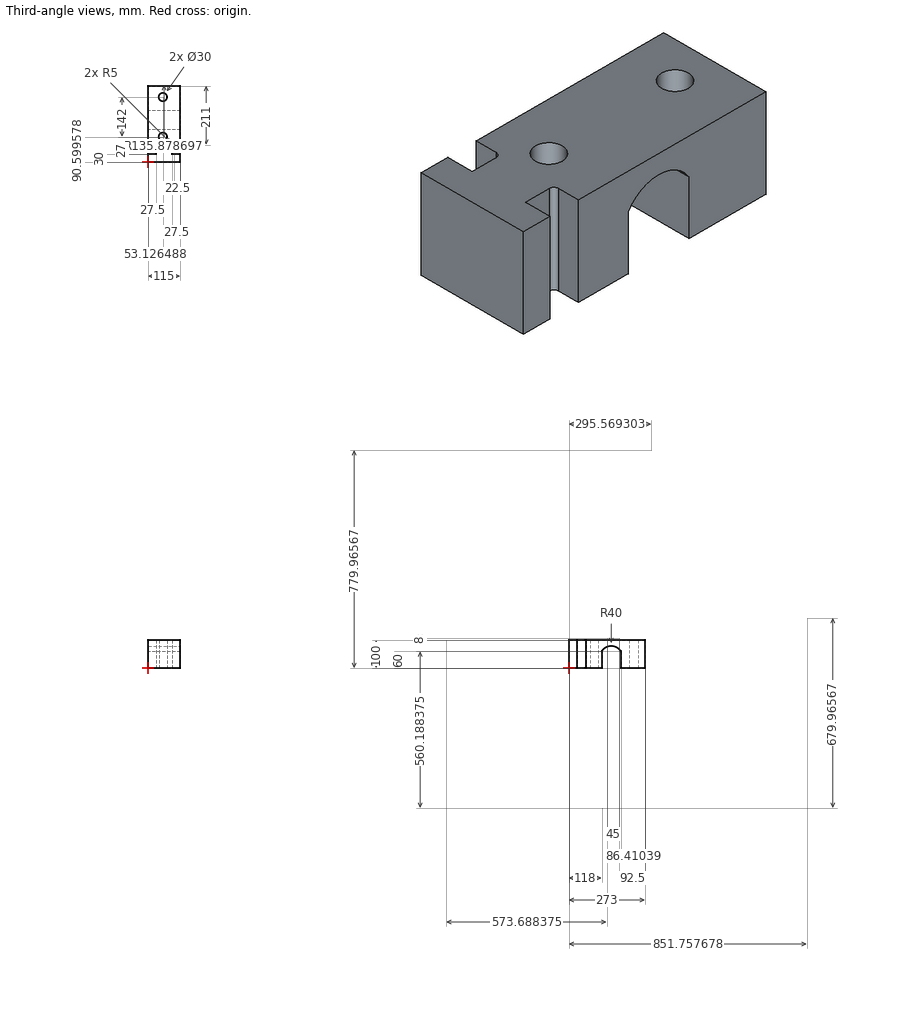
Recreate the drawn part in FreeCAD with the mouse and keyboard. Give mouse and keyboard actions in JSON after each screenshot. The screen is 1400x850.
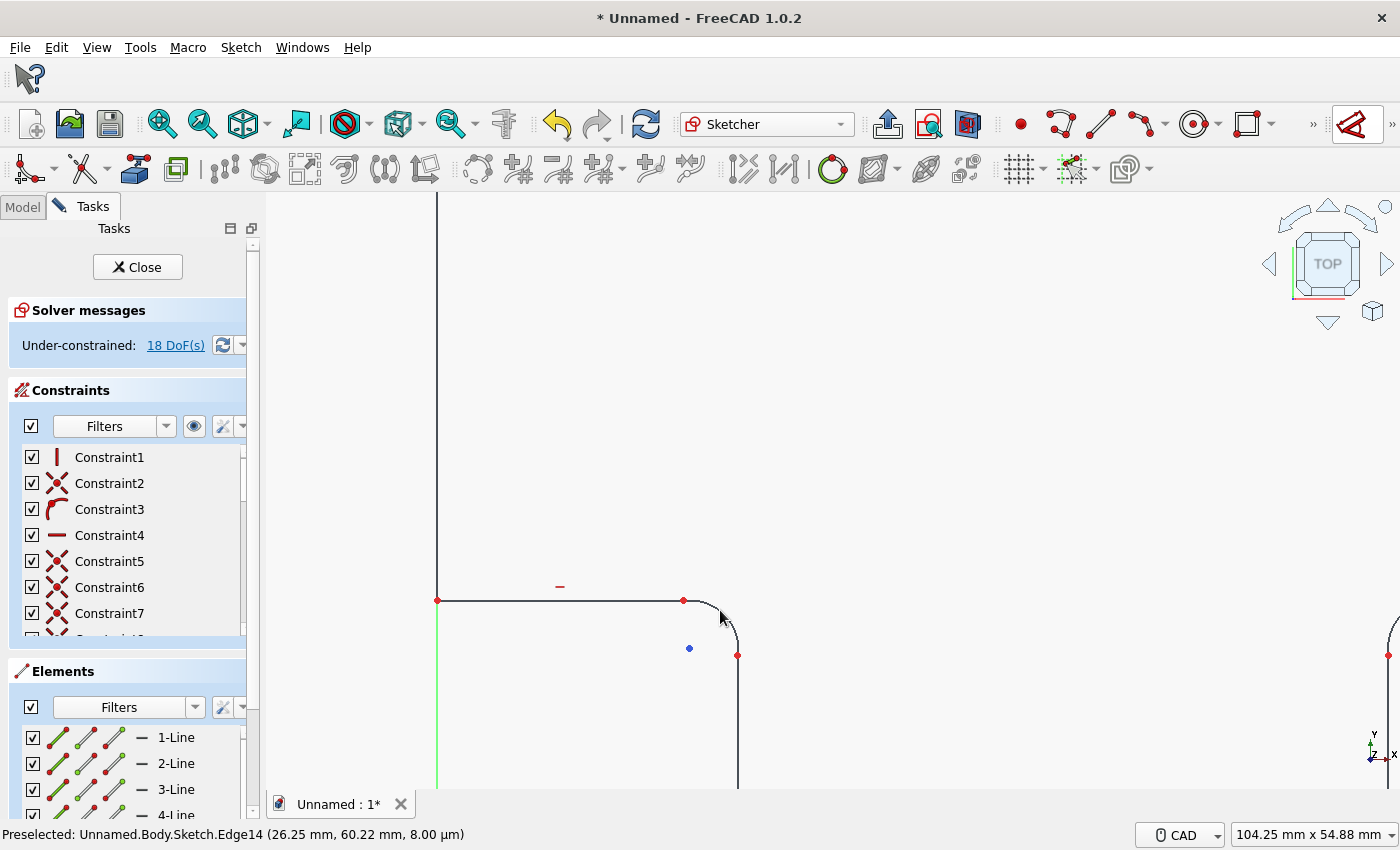
{"action": "scroll", "coordinate": [718, 612], "scroll_direction": "down", "scroll_amount": 10}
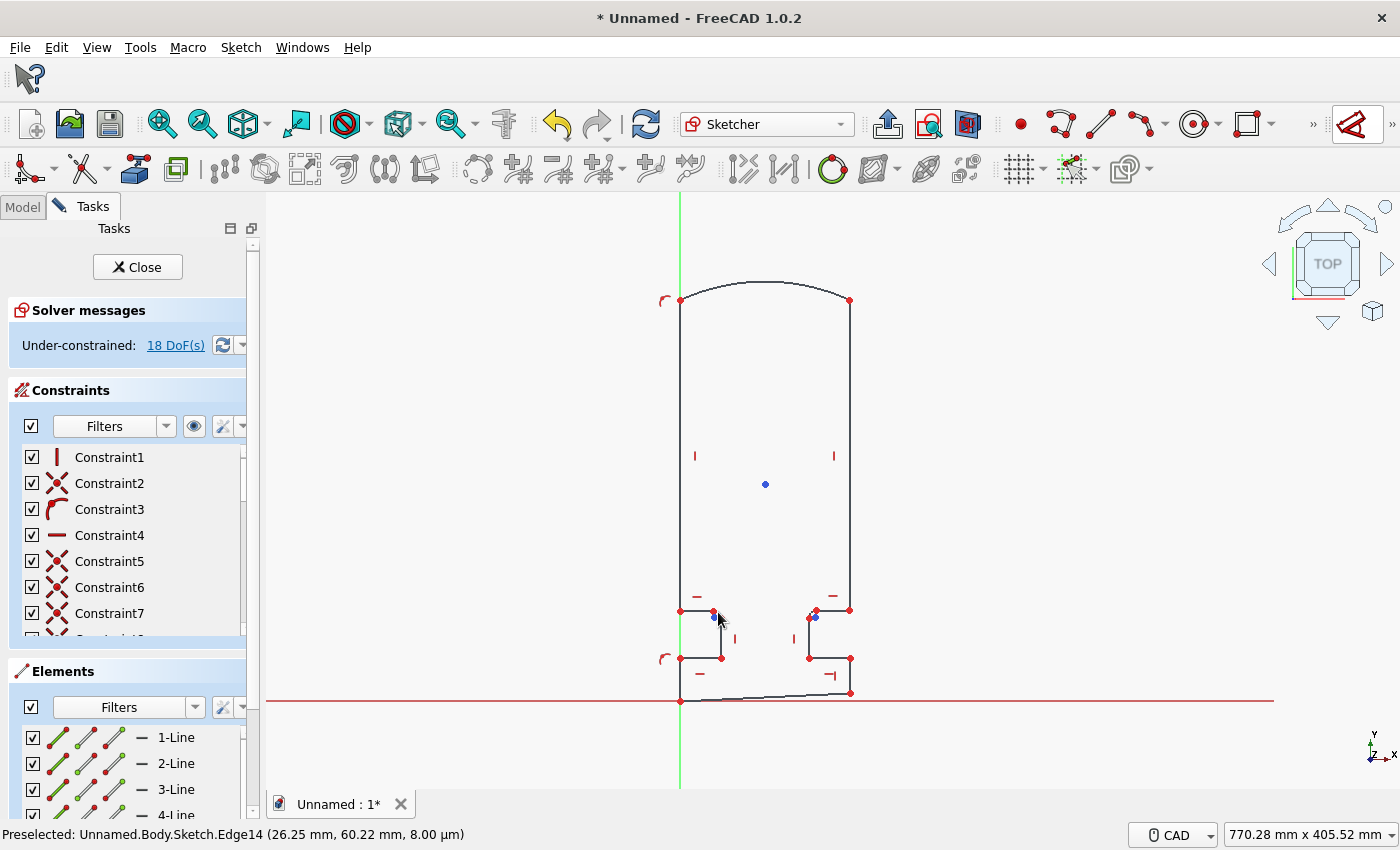
{"action": "left_click", "coordinate": [721, 630]}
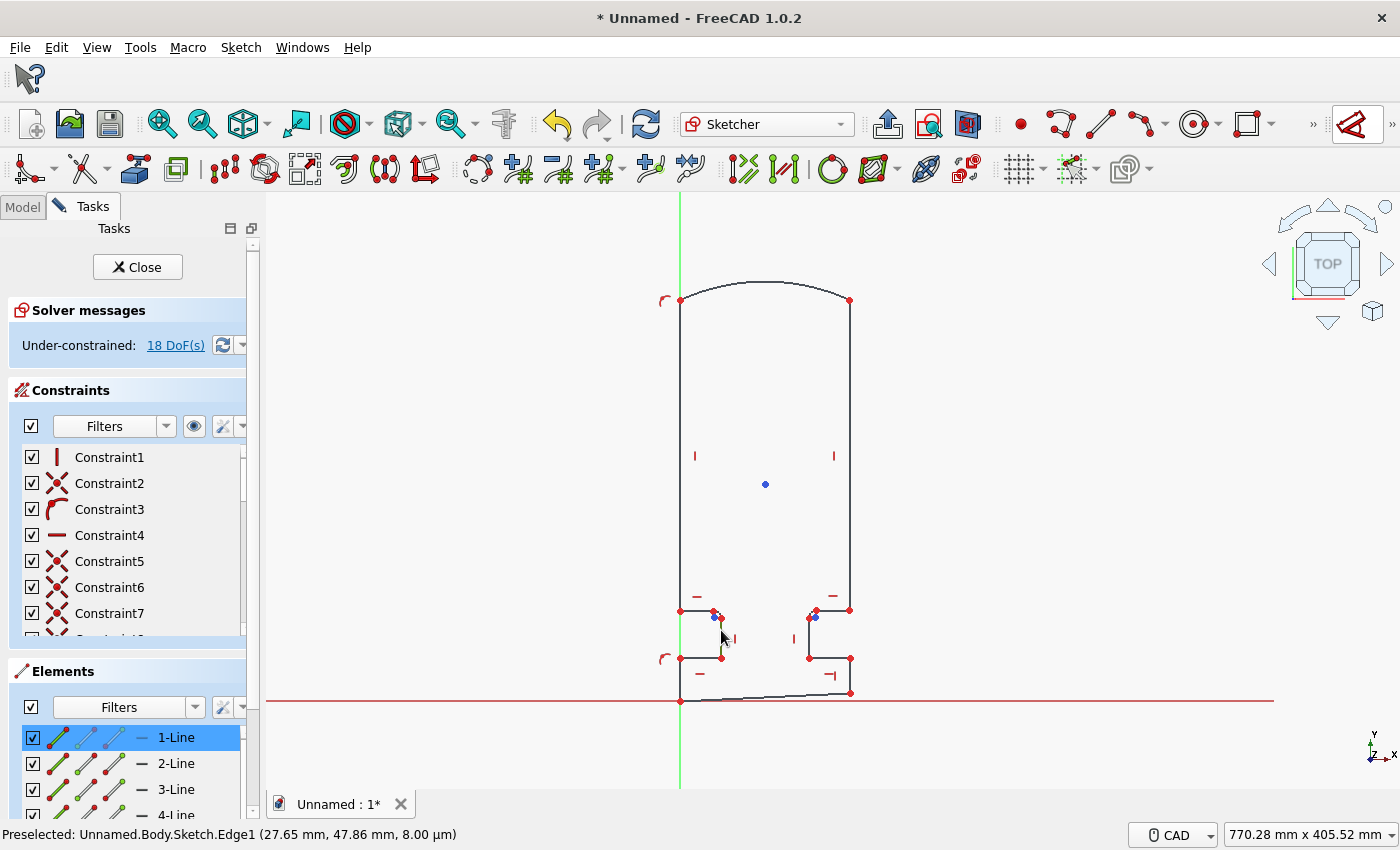
{"action": "scroll", "coordinate": [719, 613], "scroll_direction": "up", "scroll_amount": 5}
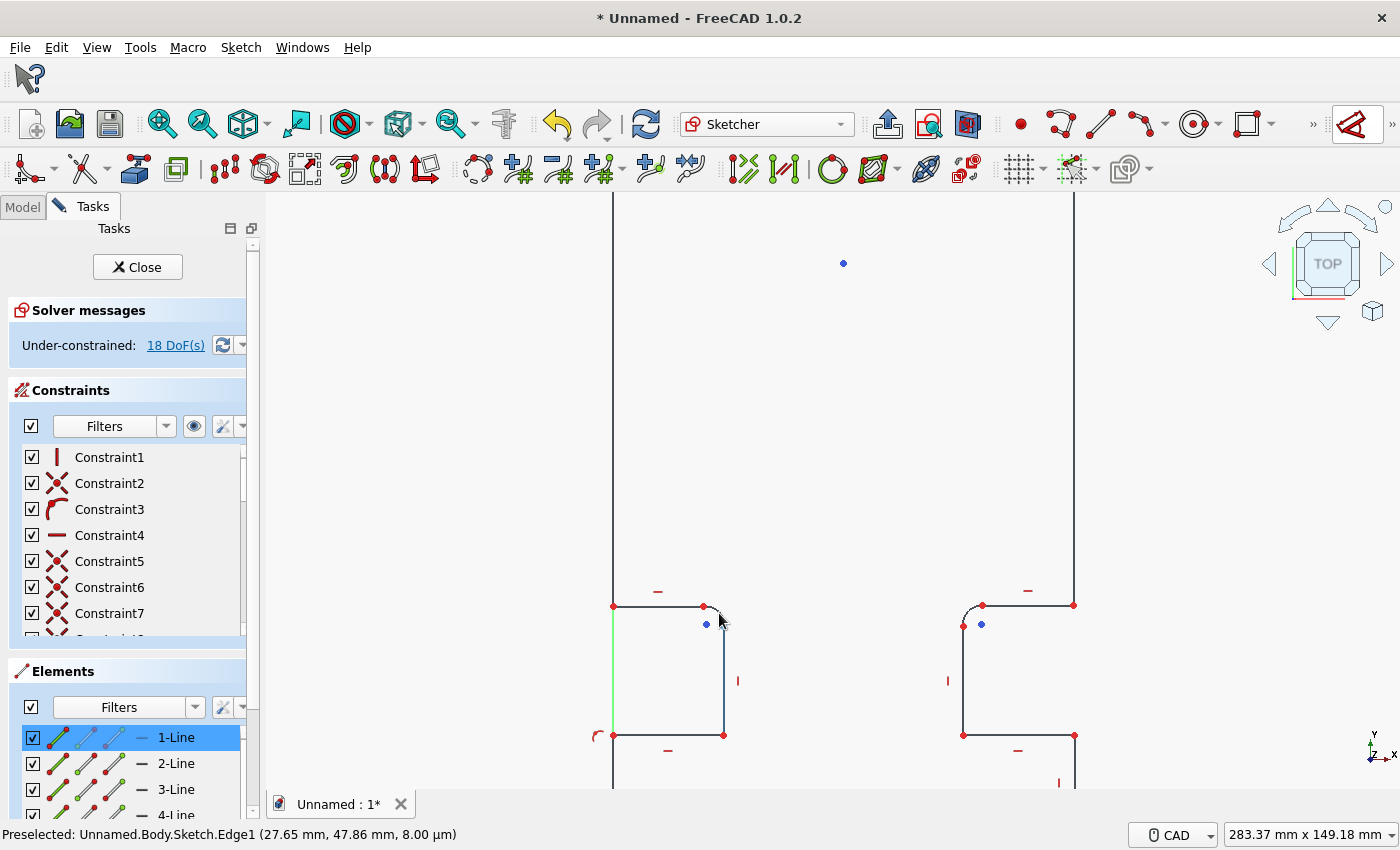
{"action": "left_click", "coordinate": [719, 612]}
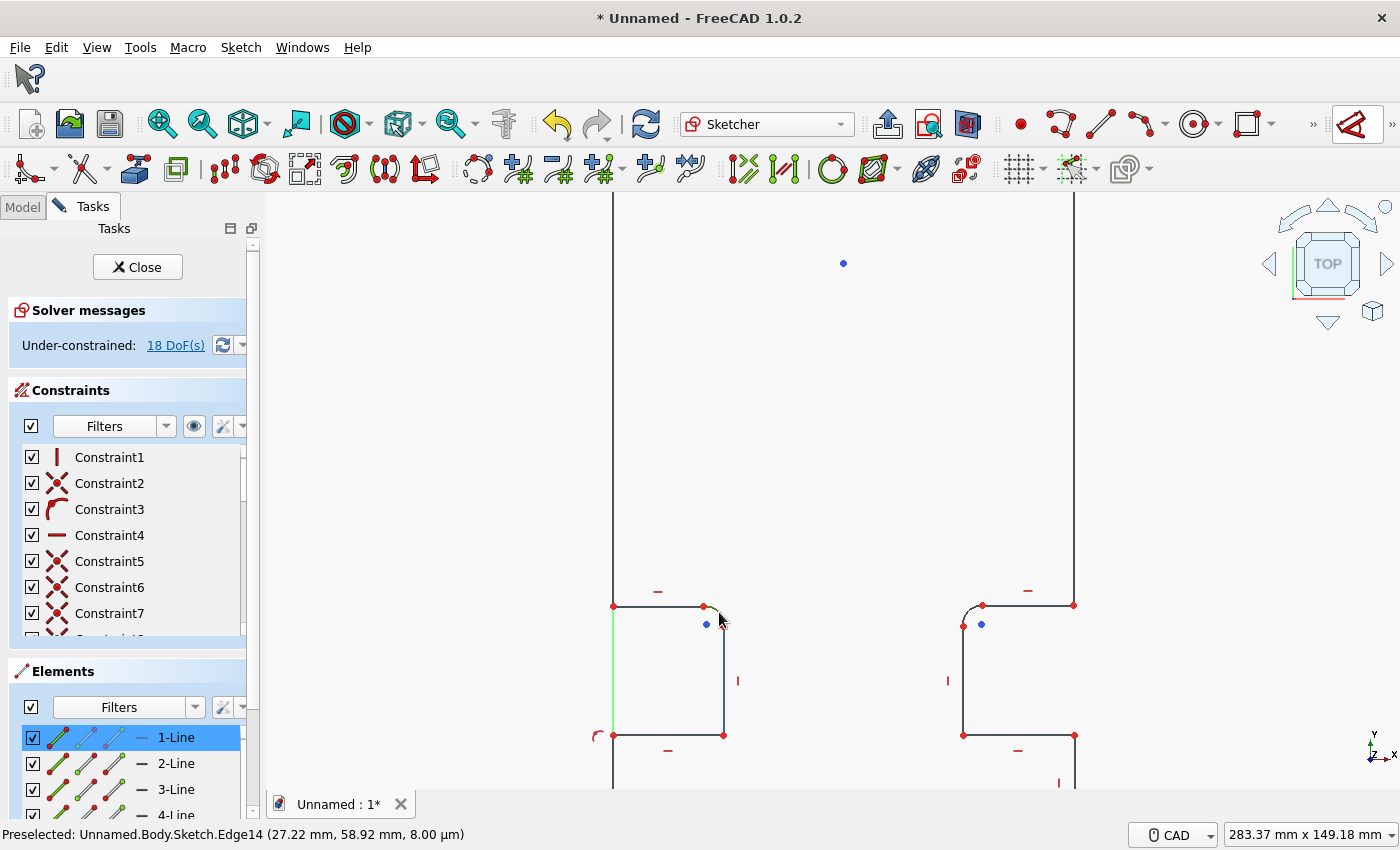
{"action": "key", "text": "t"}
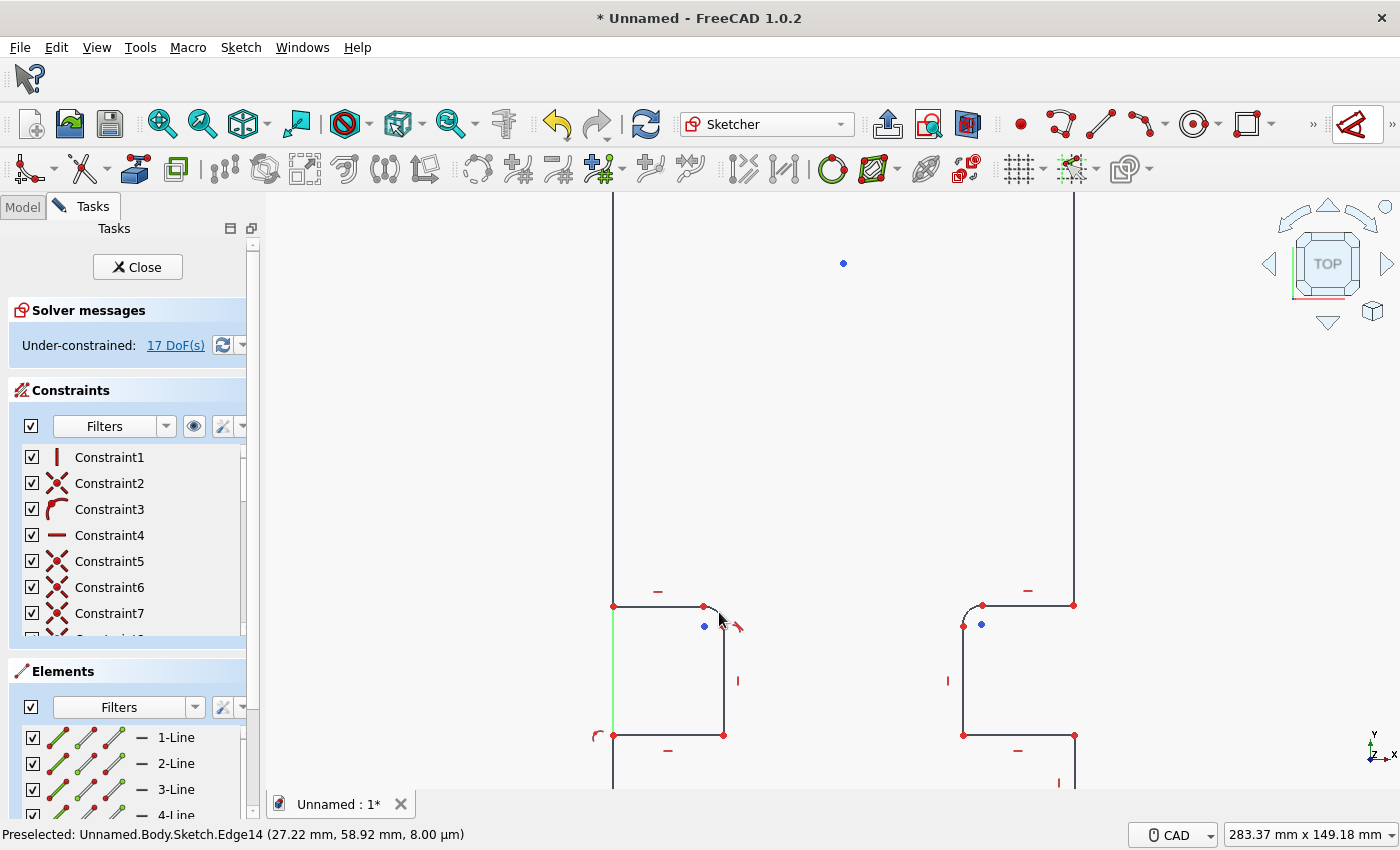
{"action": "left_click", "coordinate": [963, 703]}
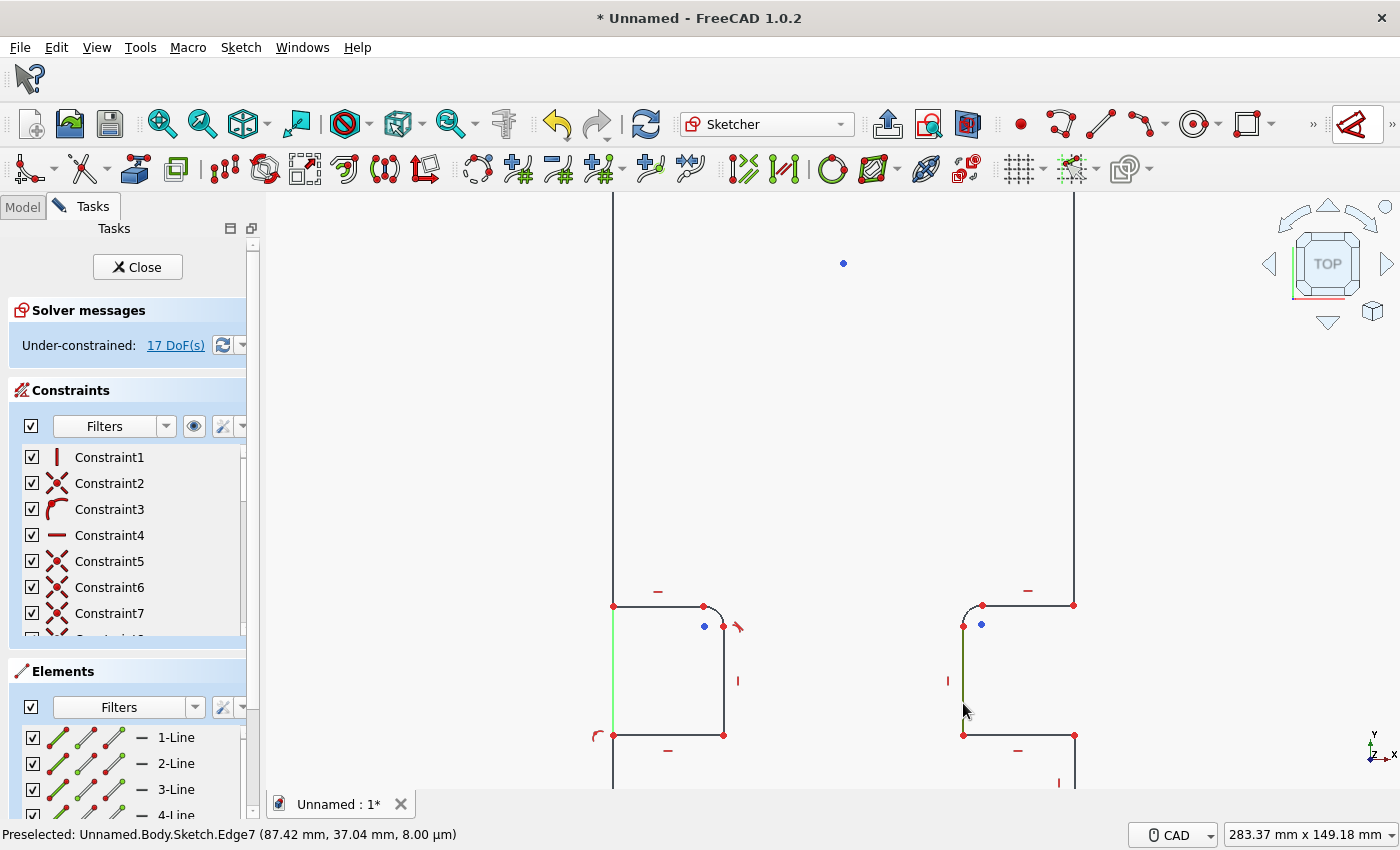
{"action": "scroll", "coordinate": [973, 608], "scroll_direction": "up", "scroll_amount": 2}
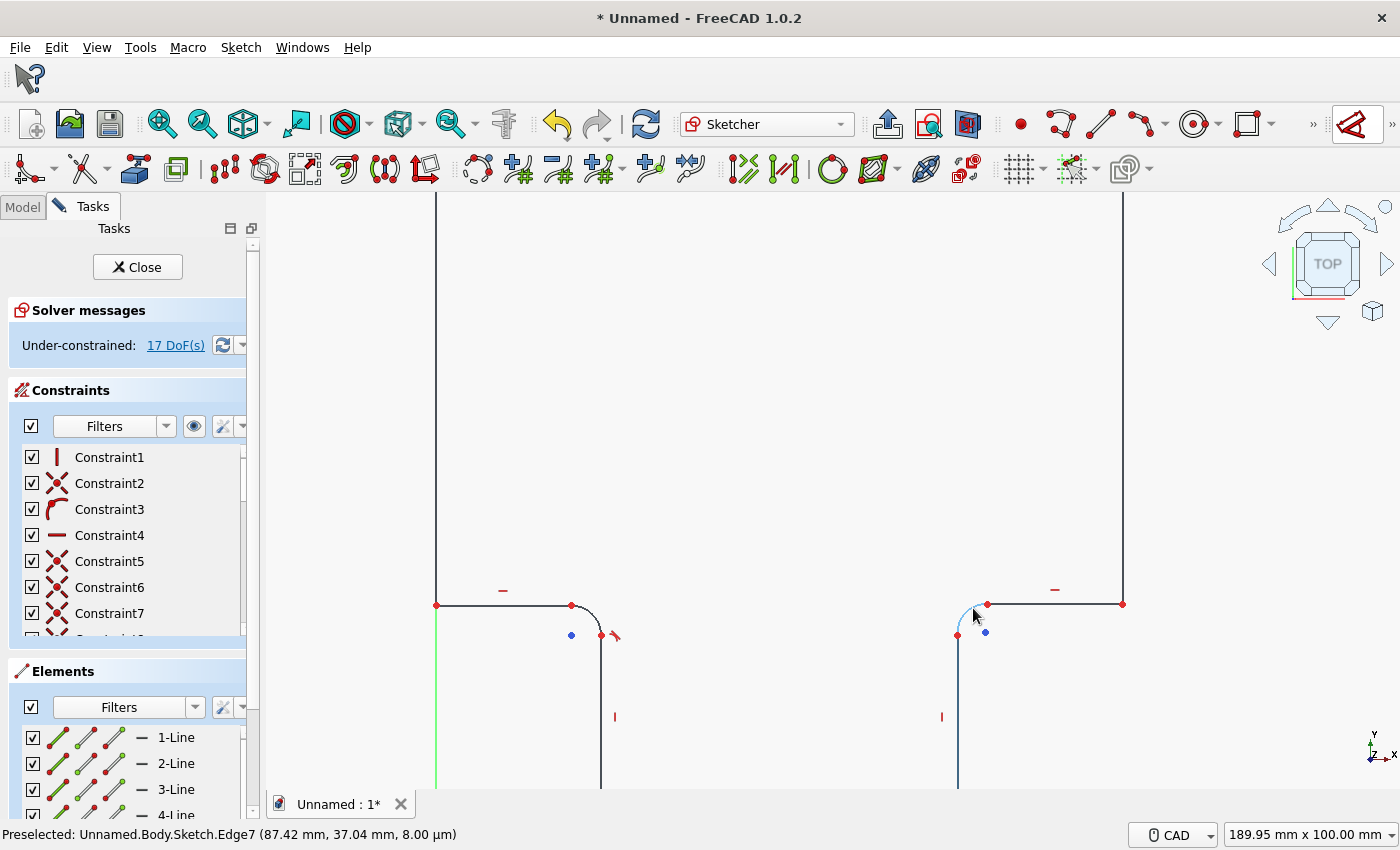
{"action": "left_click", "coordinate": [973, 607]}